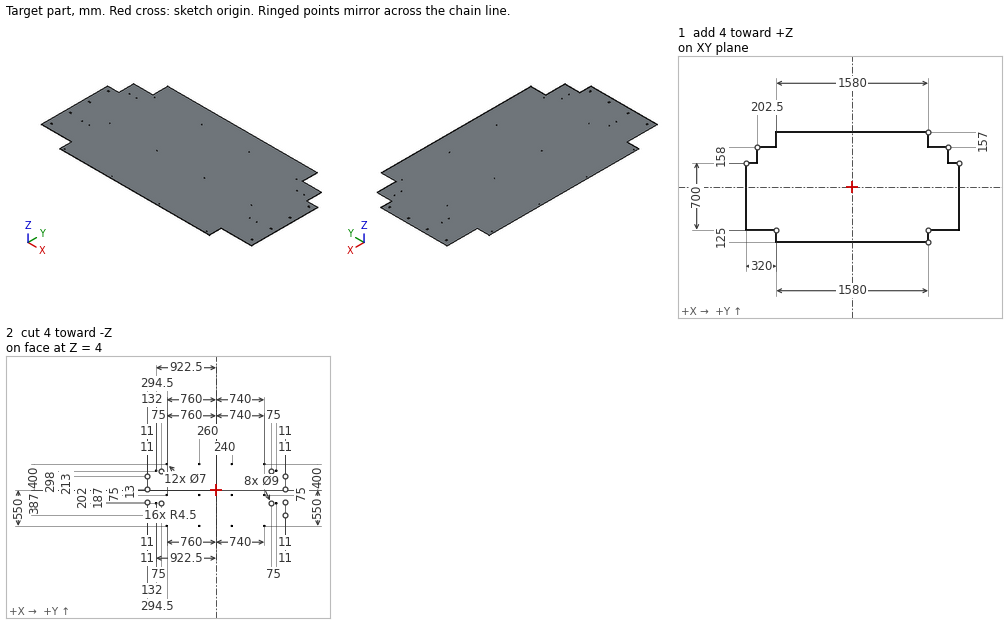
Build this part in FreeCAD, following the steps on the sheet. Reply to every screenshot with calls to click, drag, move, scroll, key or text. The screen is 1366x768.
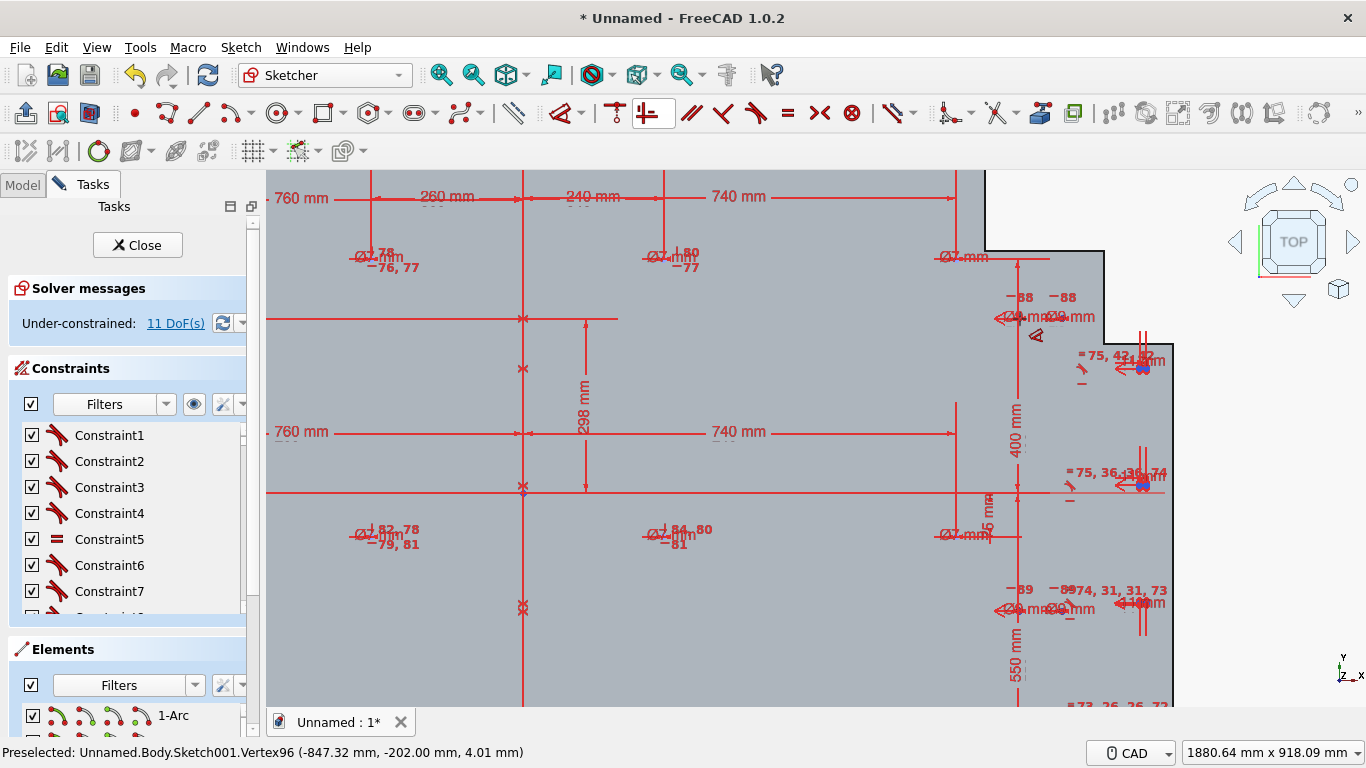
click(1019, 319)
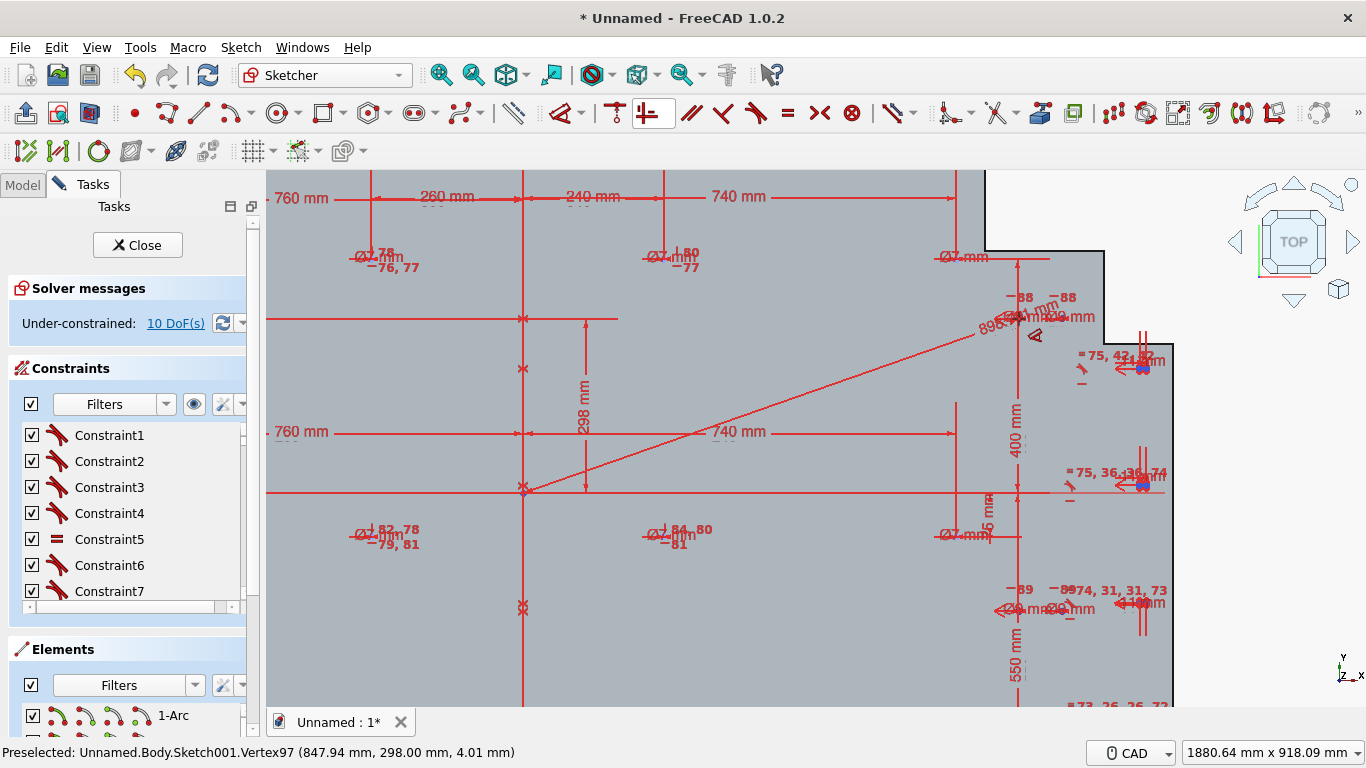
click(1062, 319)
click(1041, 285)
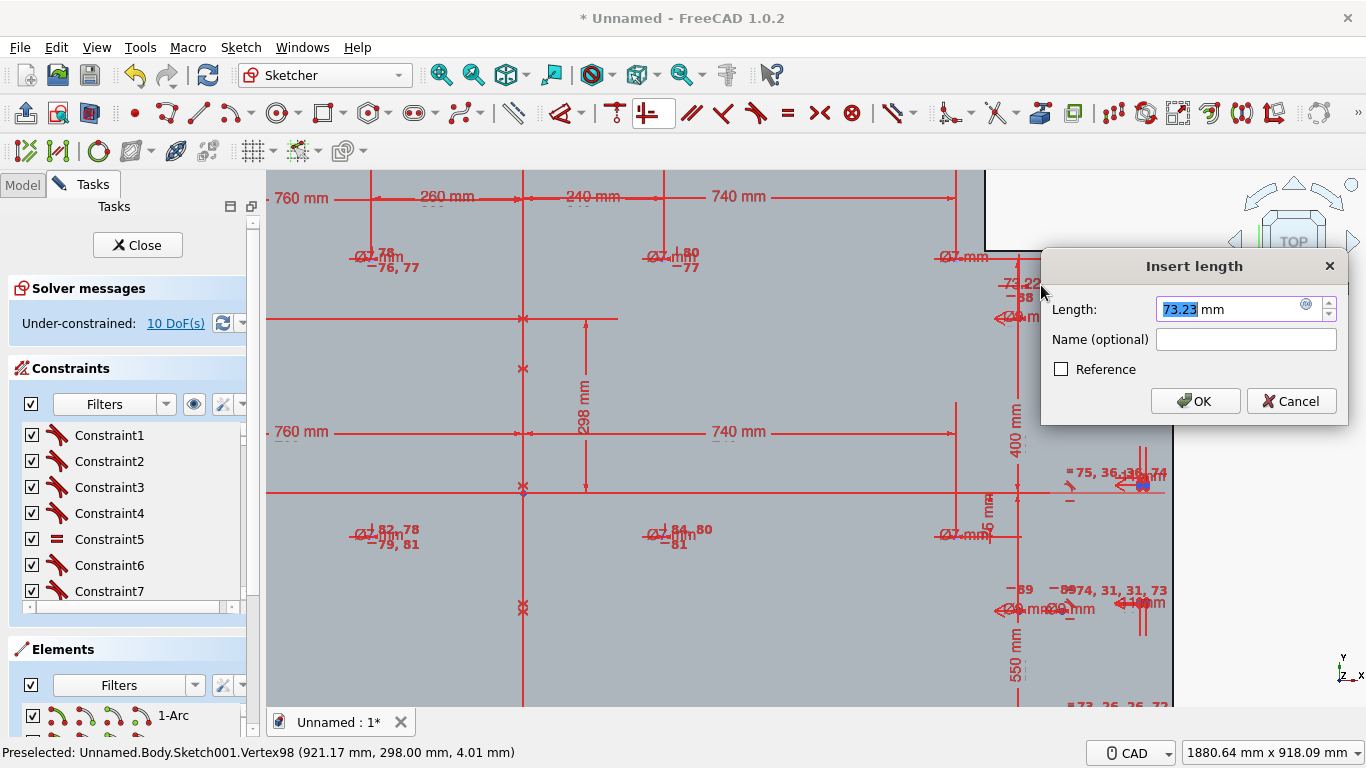
text(75)
key(Return)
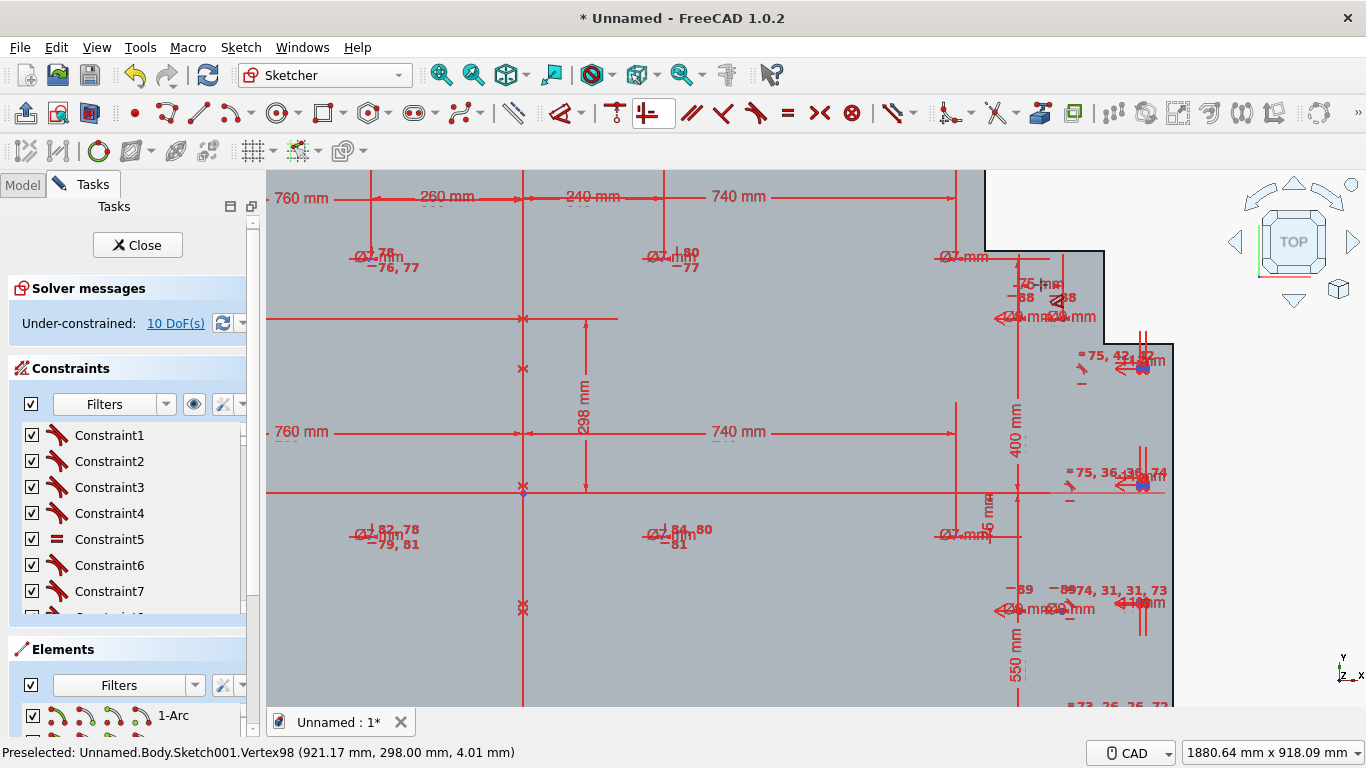
click(1019, 611)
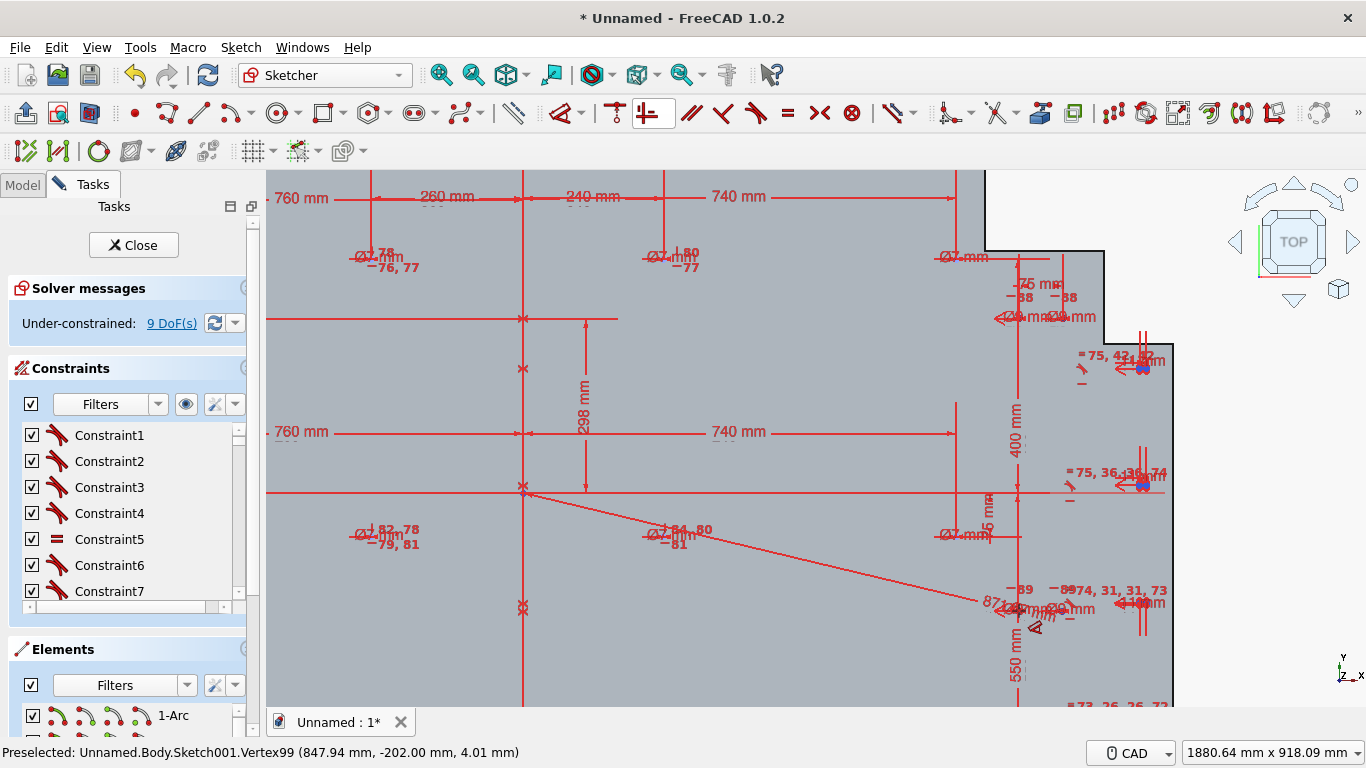
click(1062, 611)
click(1041, 577)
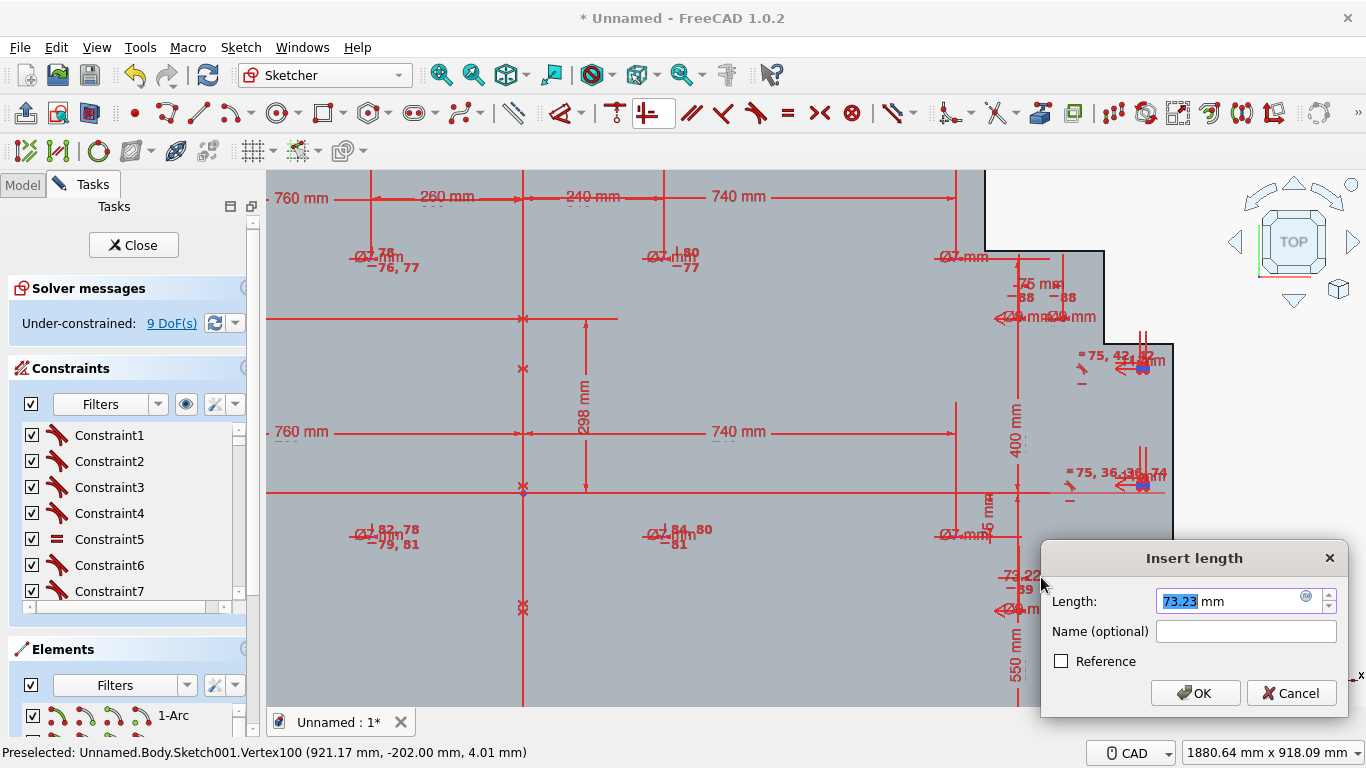
text(75)
key(Return)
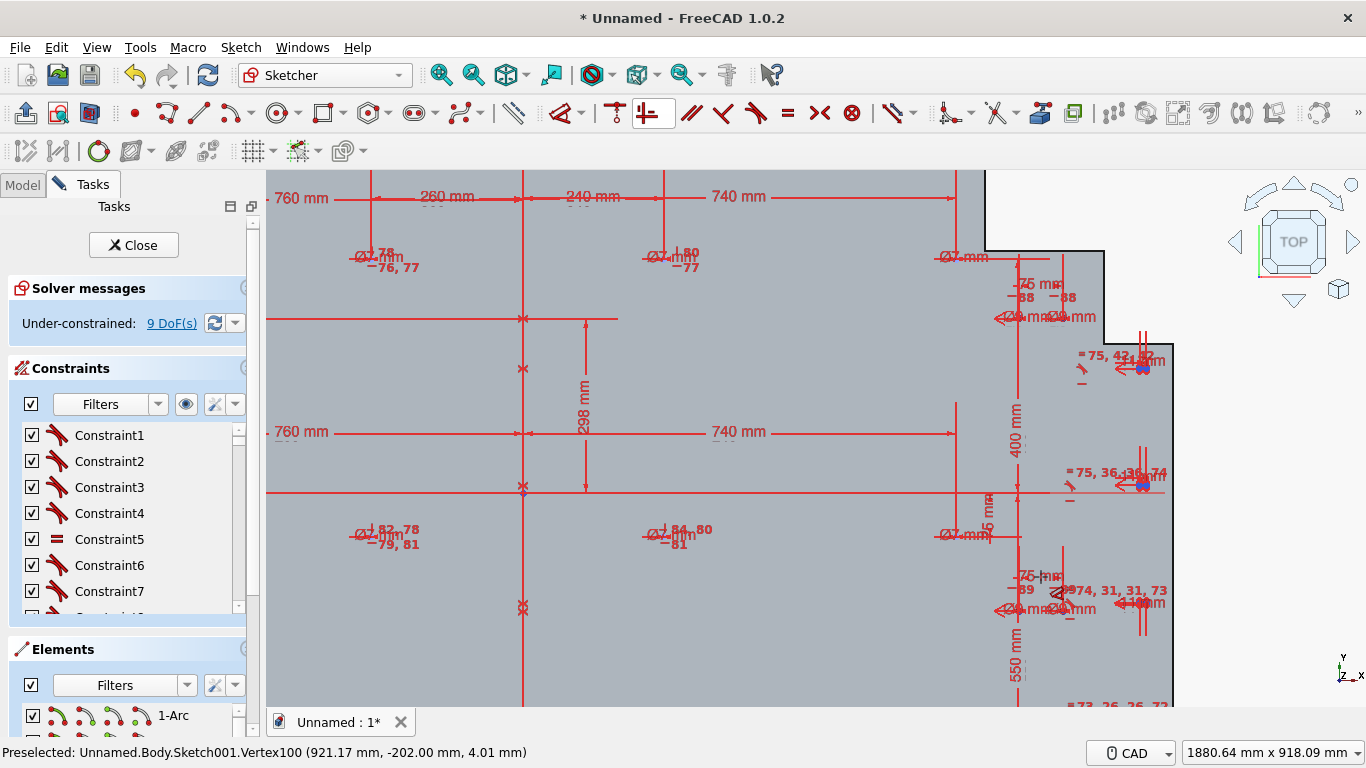
scroll(1020, 319, down, 3)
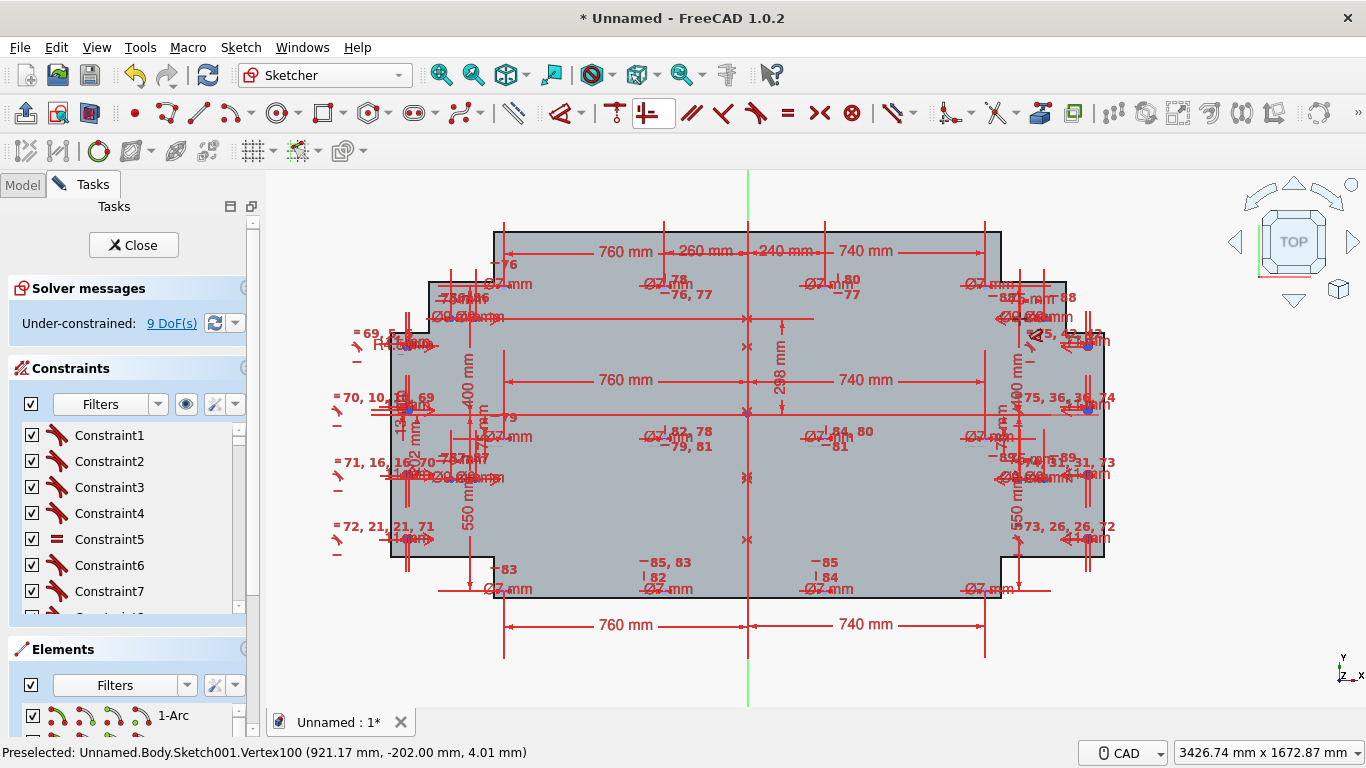
scroll(406, 347, up, 11)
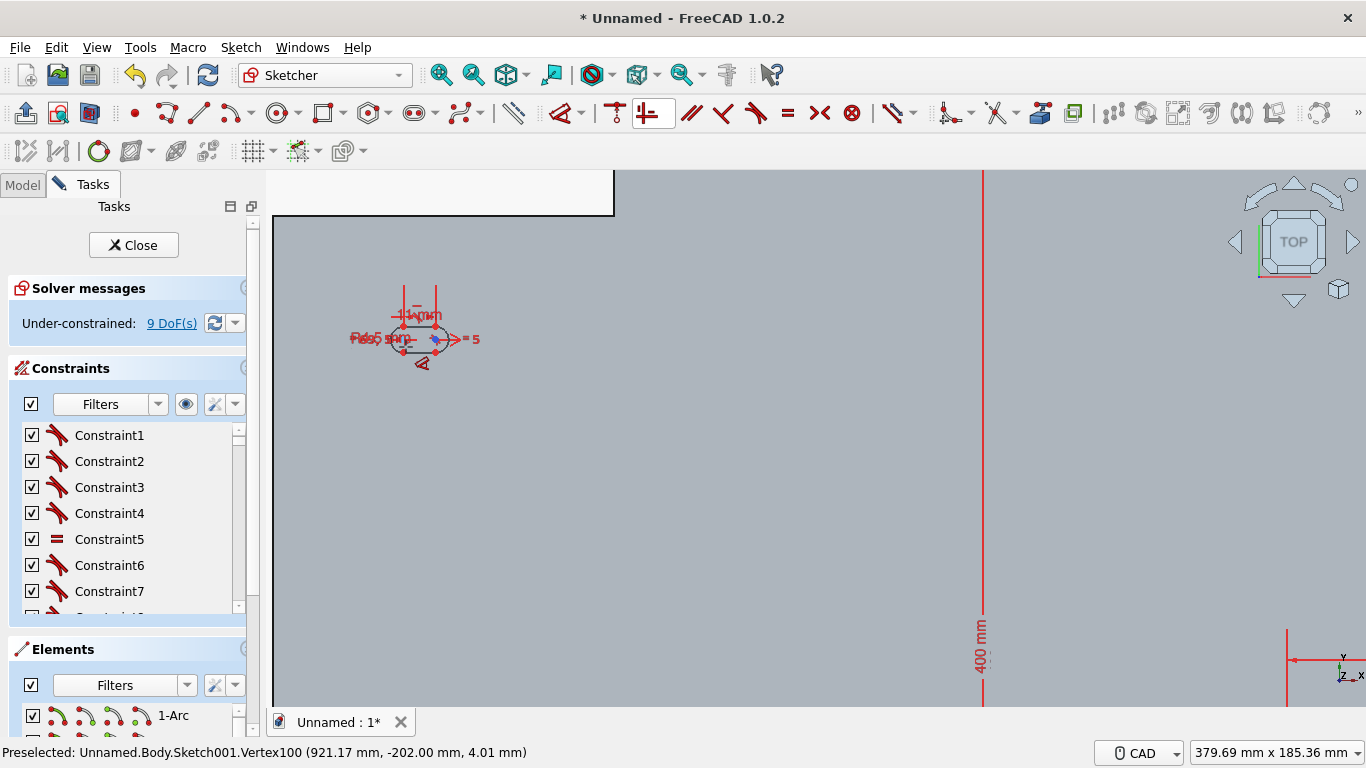
click(404, 340)
click(370, 509)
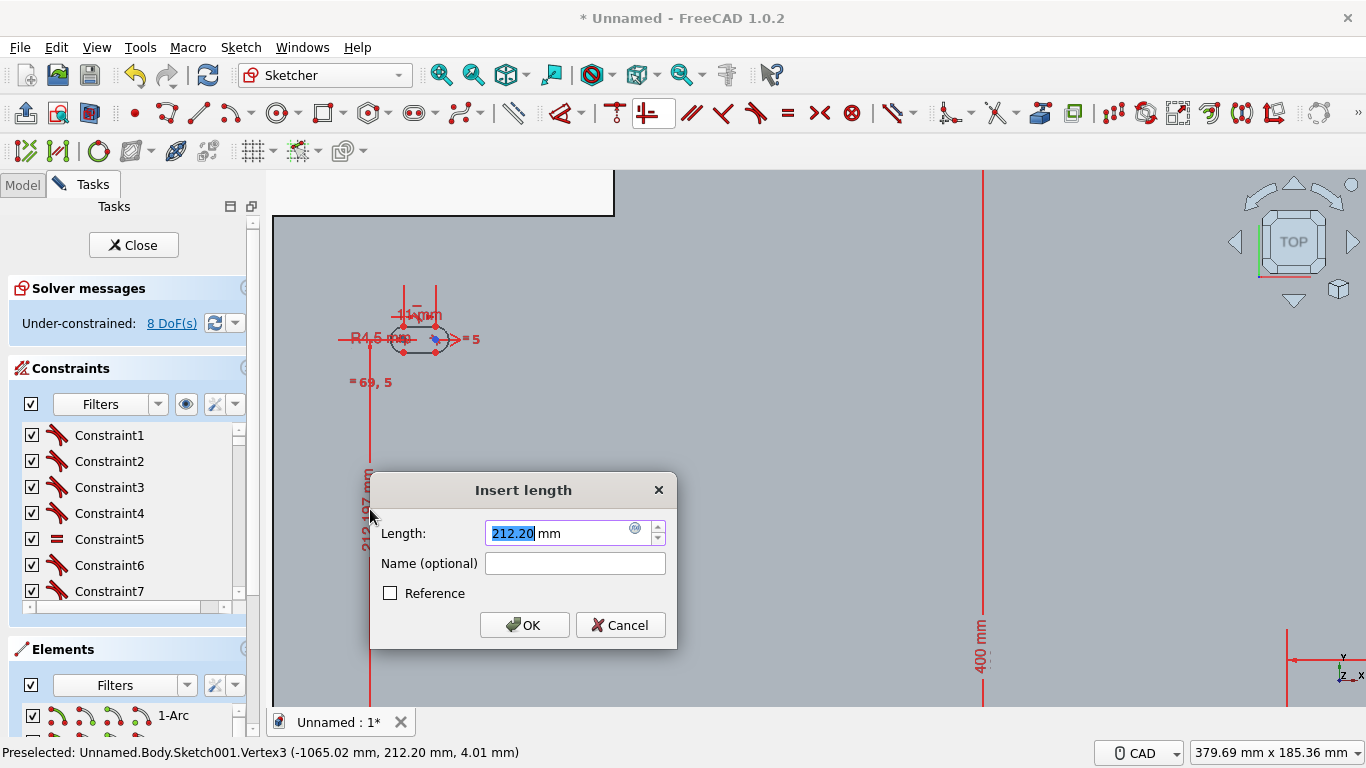
text(213)
key(Return)